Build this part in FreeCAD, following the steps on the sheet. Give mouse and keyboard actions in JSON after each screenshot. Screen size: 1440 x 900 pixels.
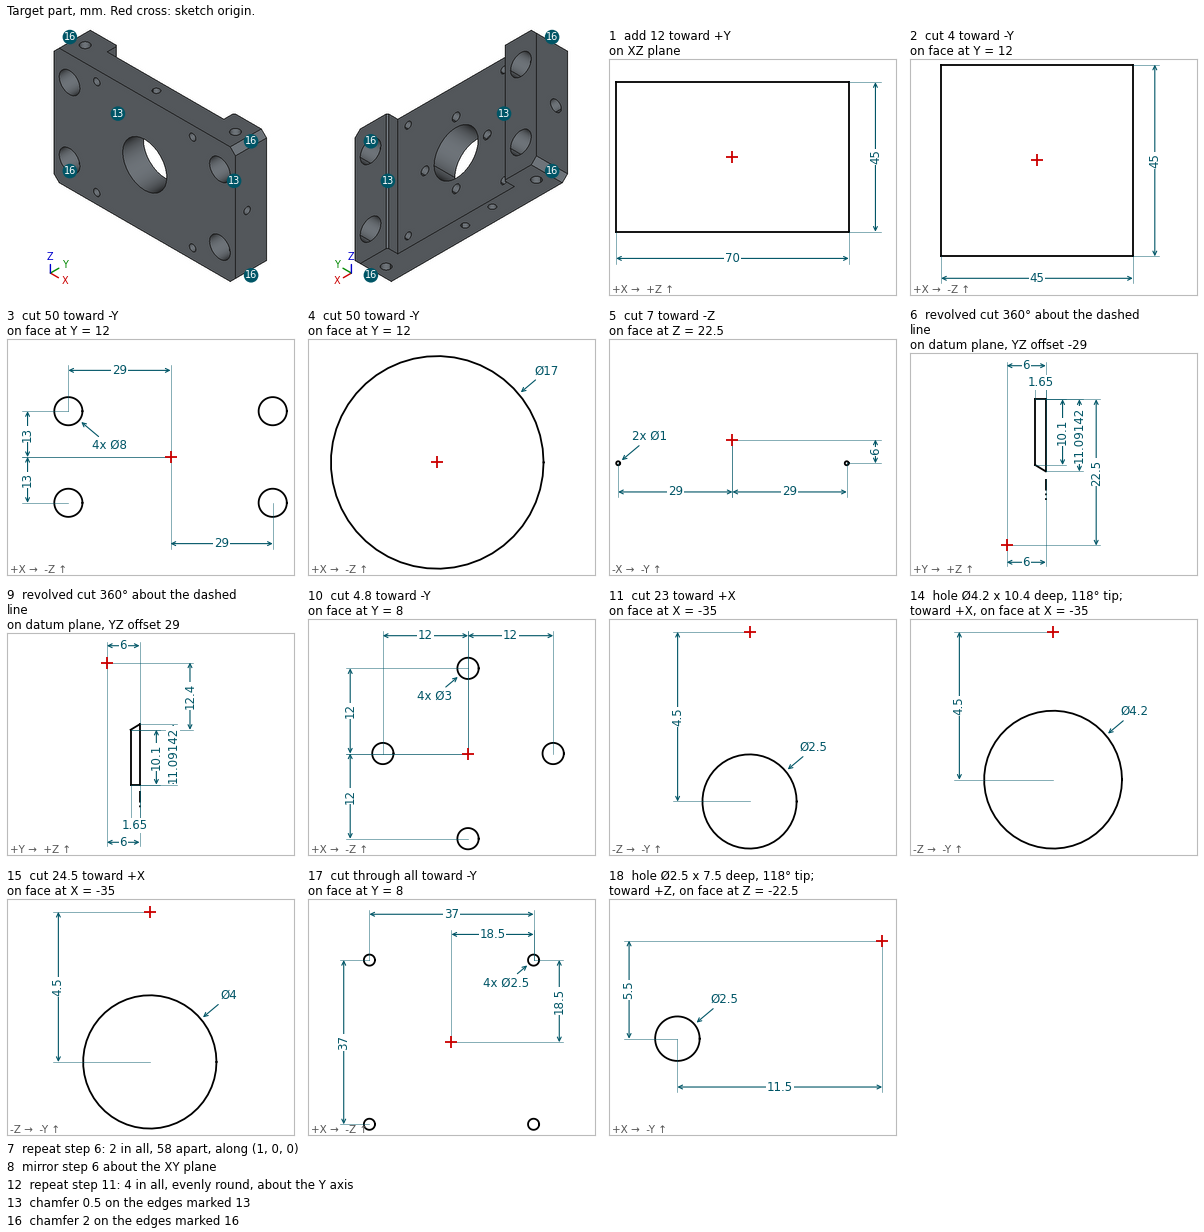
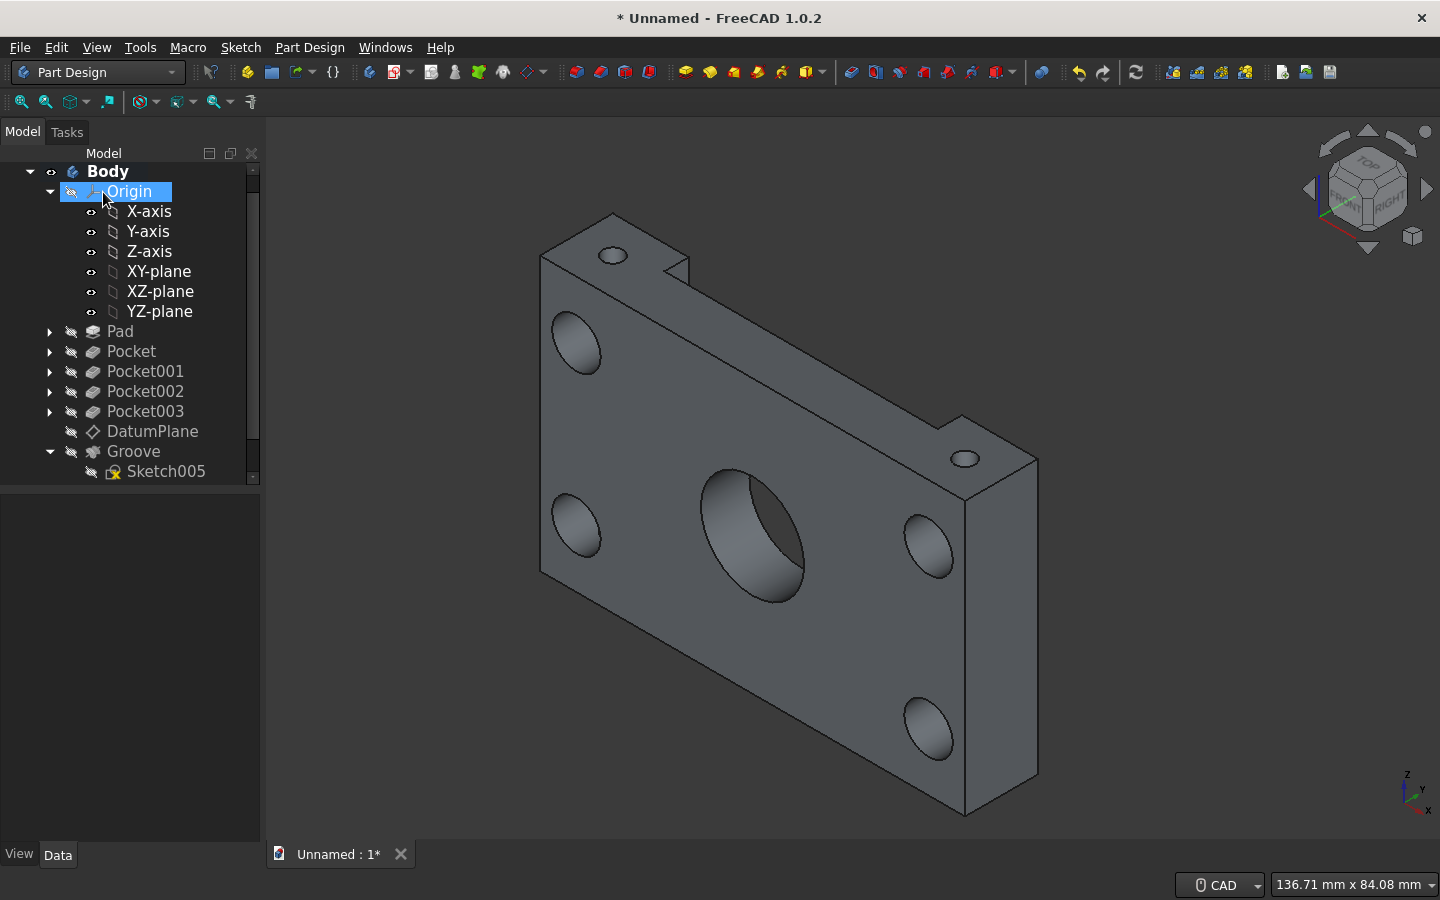
{"action": "left_click", "coordinate": [136, 312]}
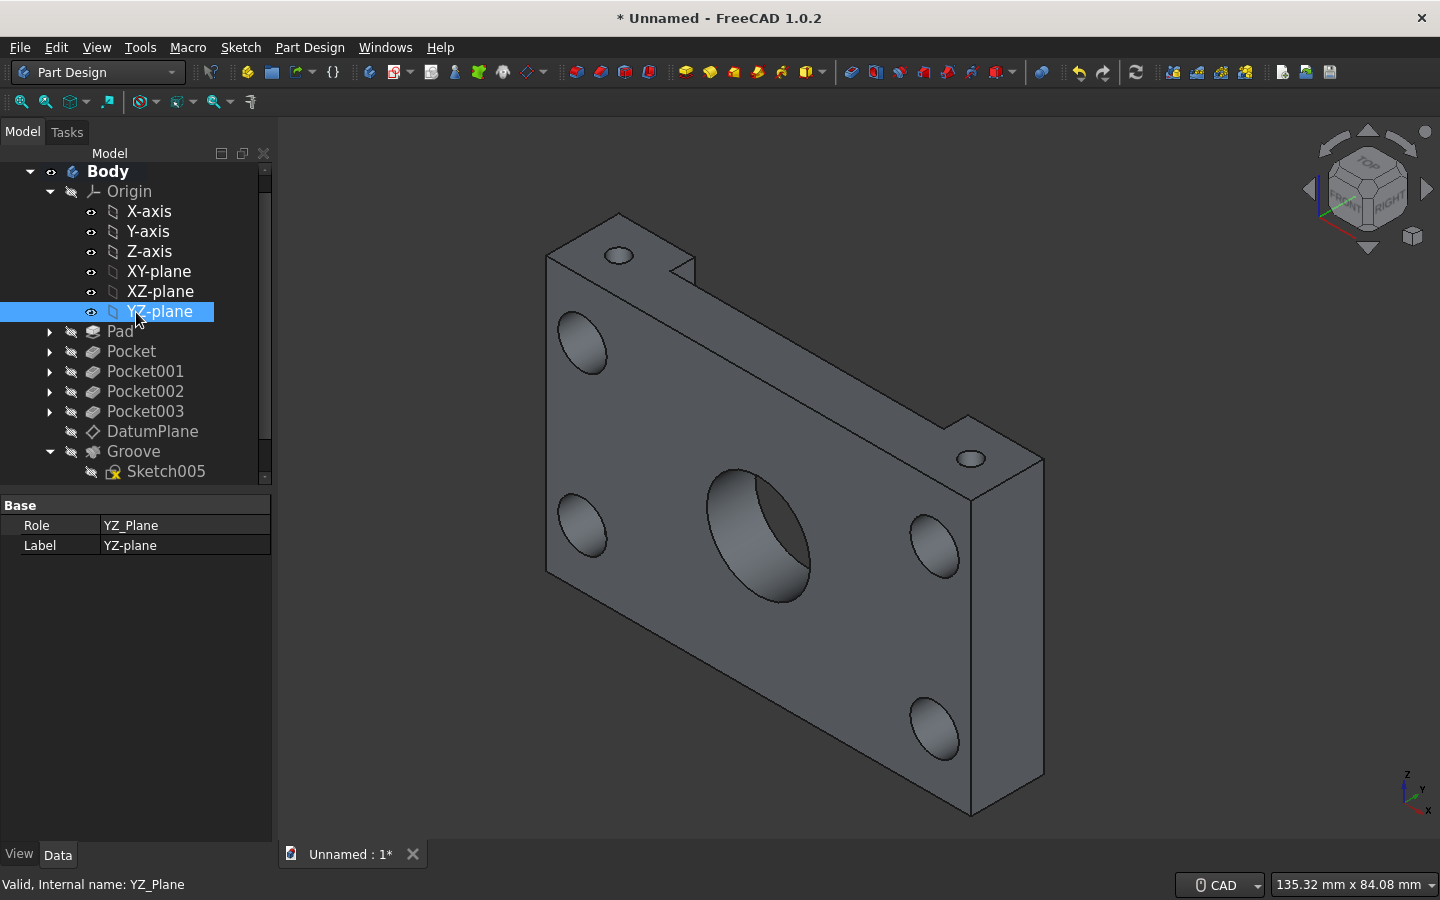
{"action": "left_click", "coordinate": [528, 72]}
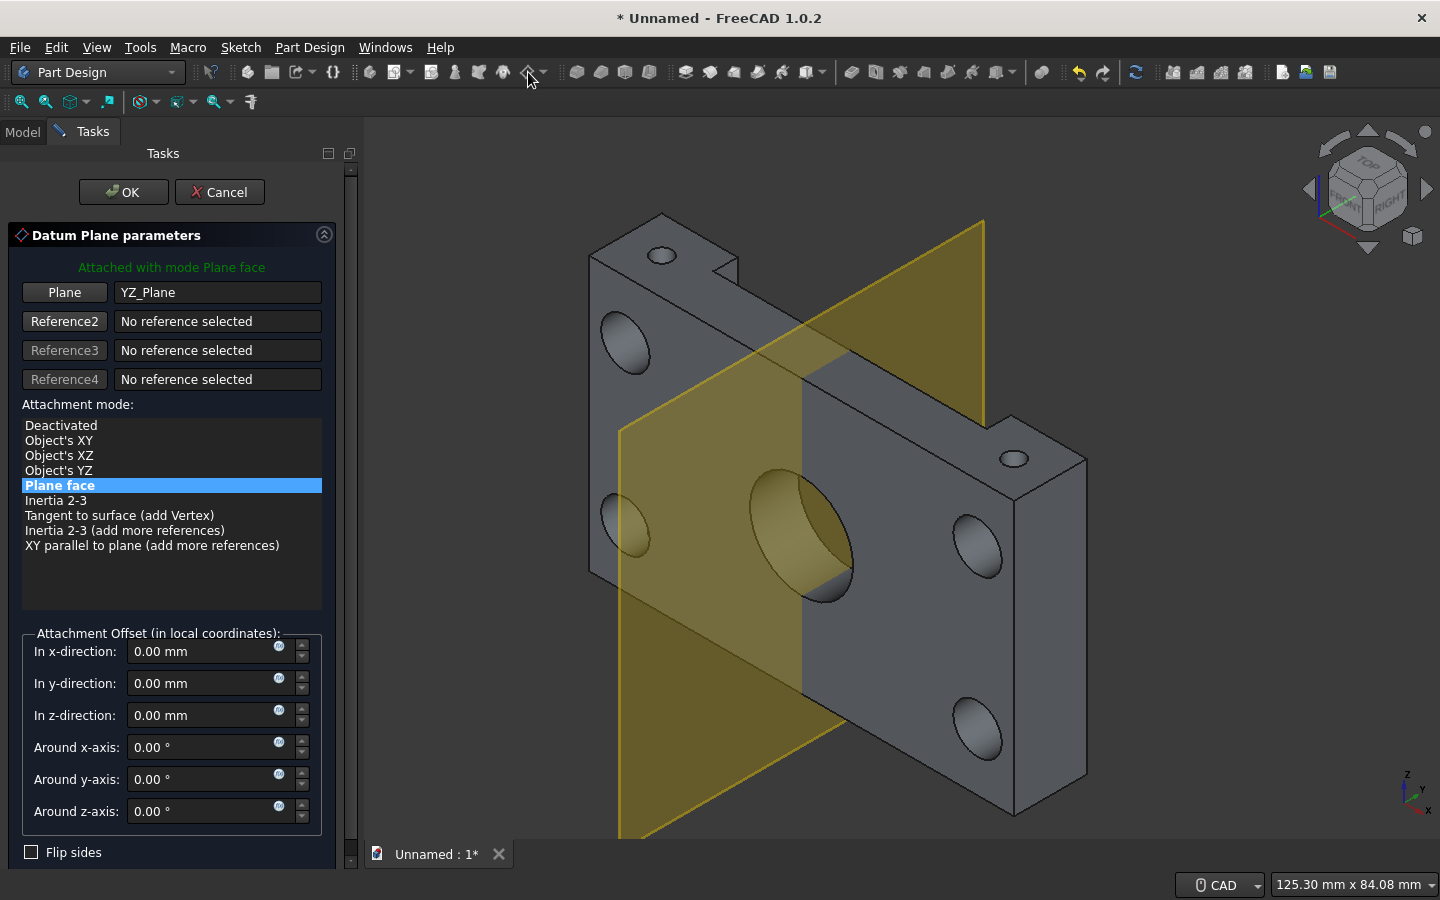
{"action": "triple_click", "coordinate": [210, 715]}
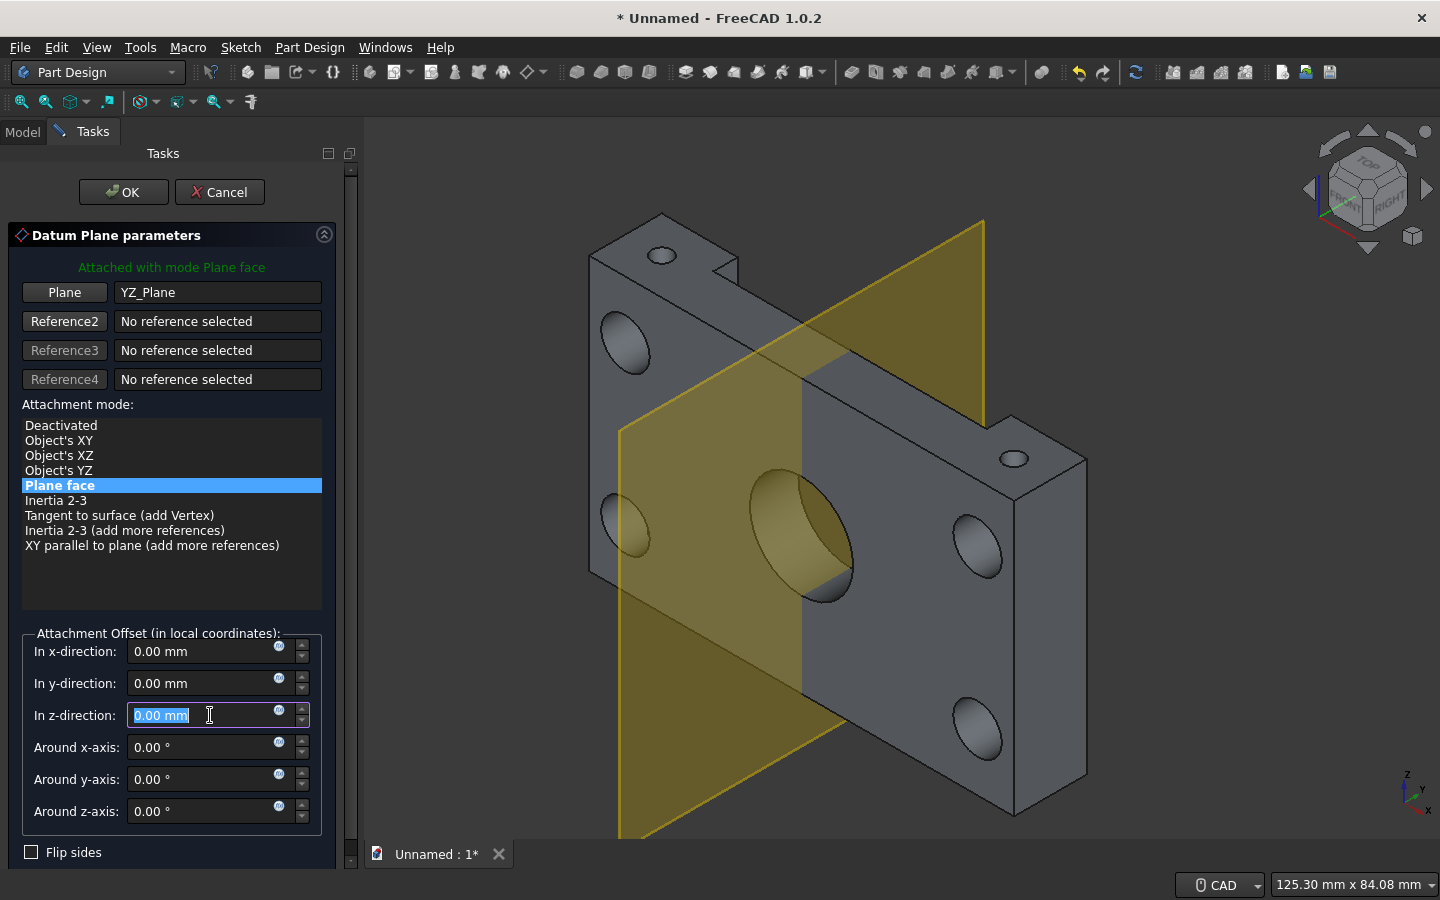
{"action": "type", "text": "29"}
{"action": "key", "text": "Tab"}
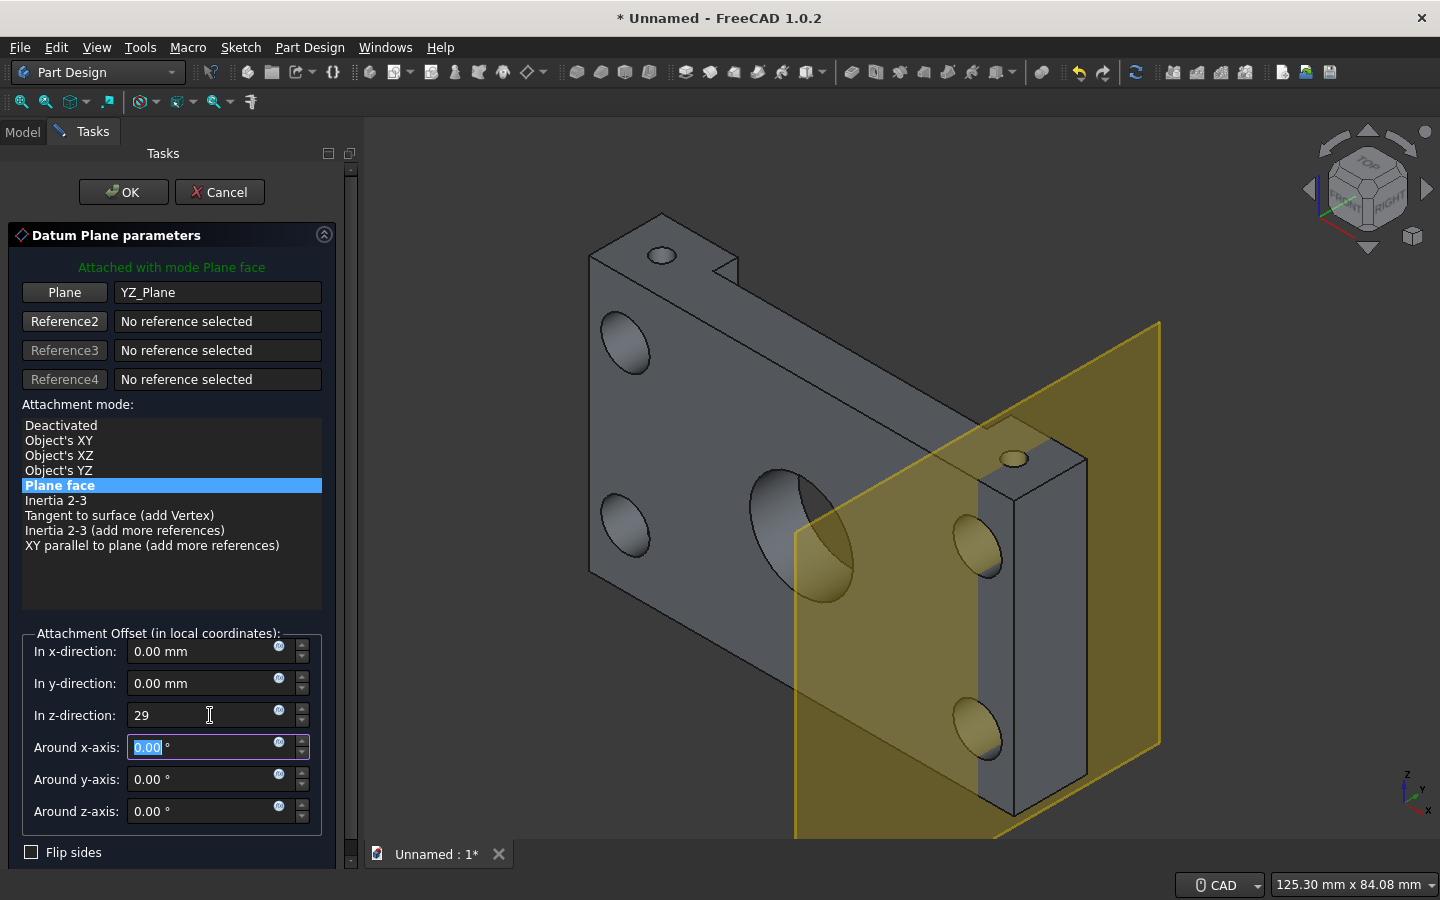
{"action": "left_click", "coordinate": [124, 192]}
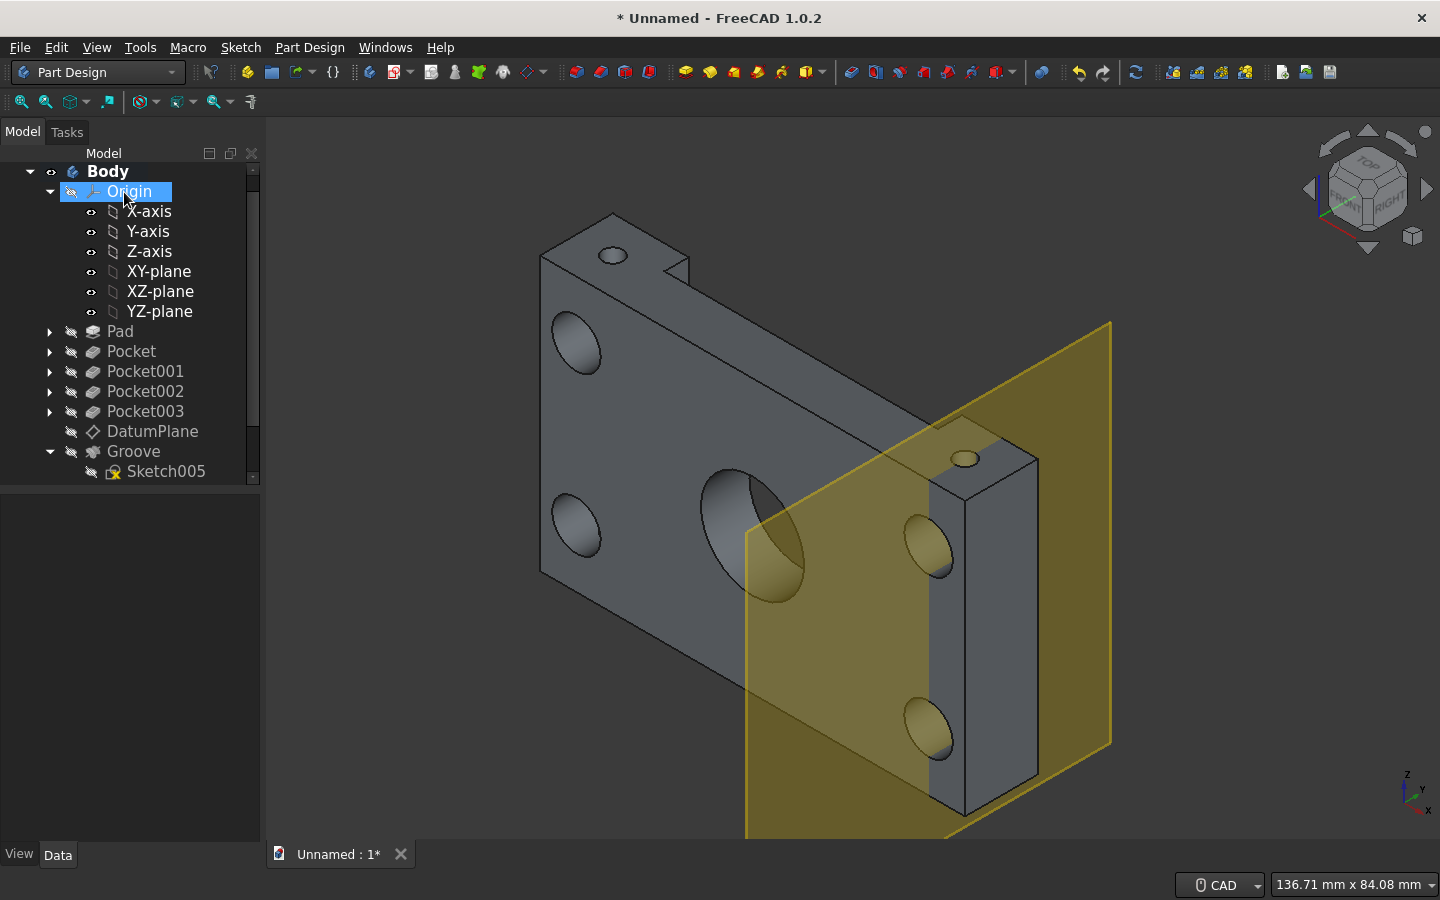
{"action": "scroll", "coordinate": [120, 327], "scroll_direction": "down", "scroll_amount": 3}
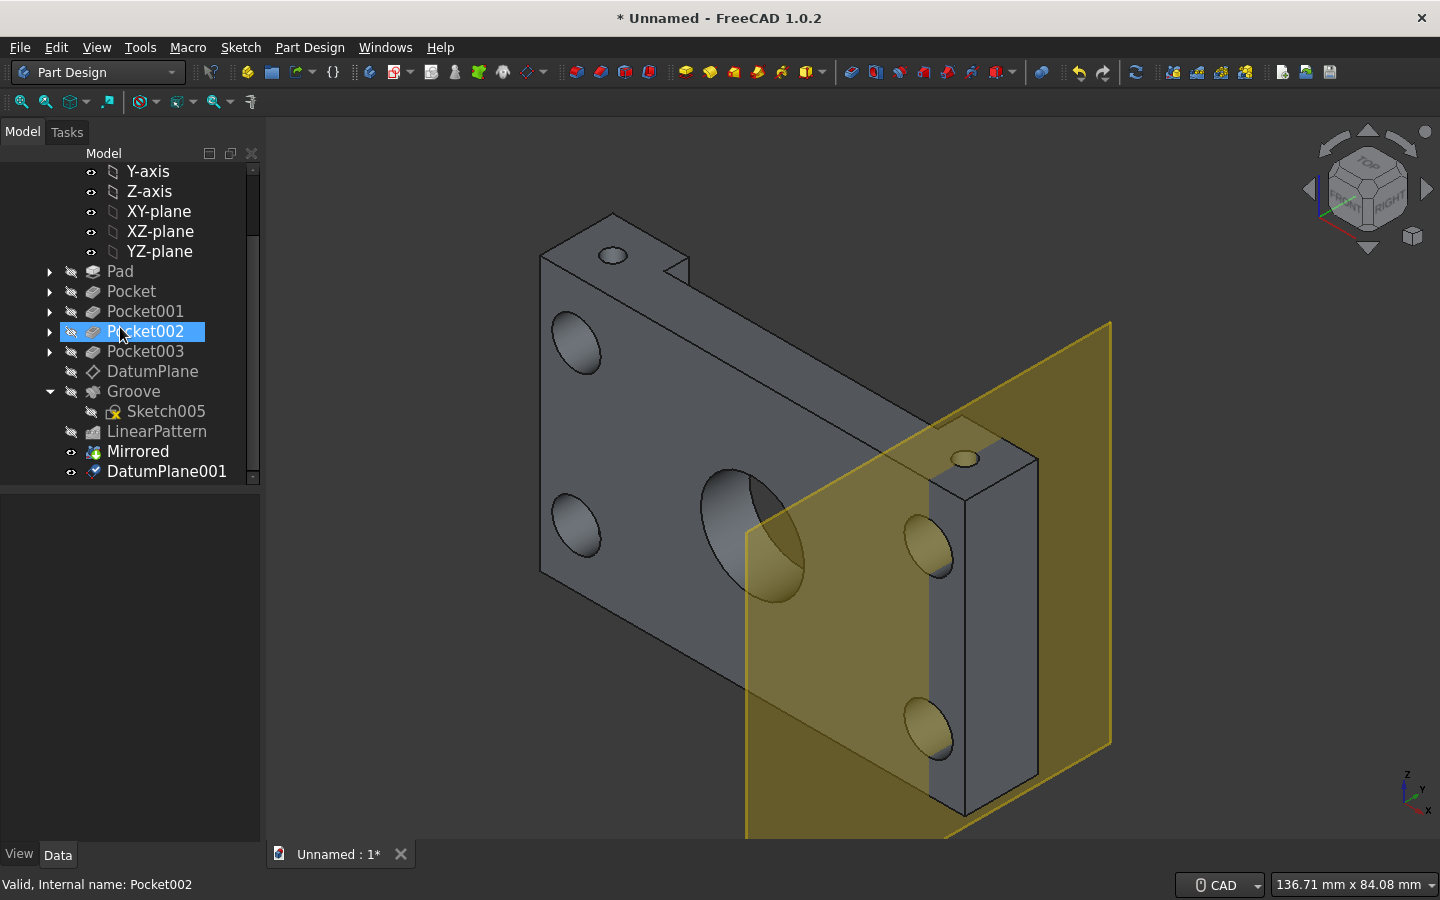
{"action": "left_click", "coordinate": [116, 472]}